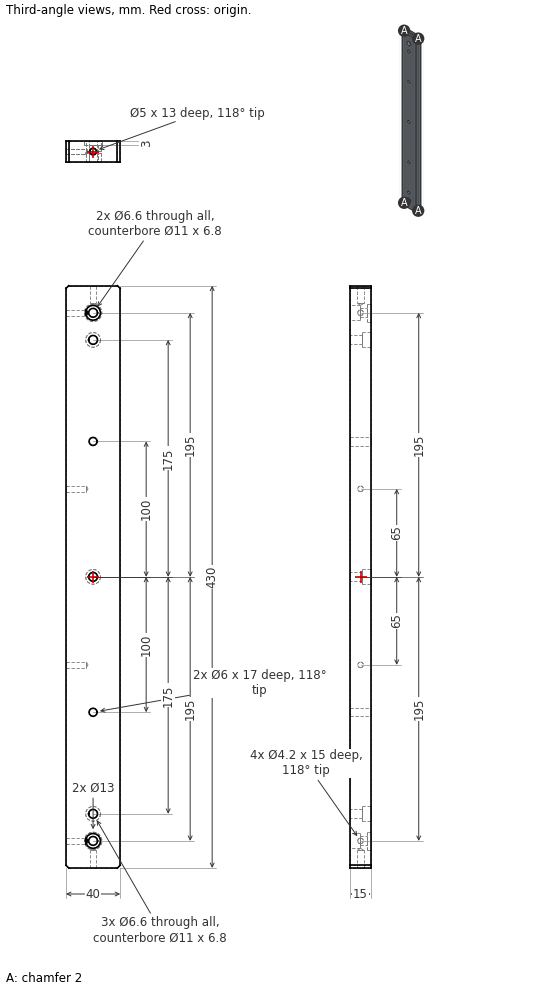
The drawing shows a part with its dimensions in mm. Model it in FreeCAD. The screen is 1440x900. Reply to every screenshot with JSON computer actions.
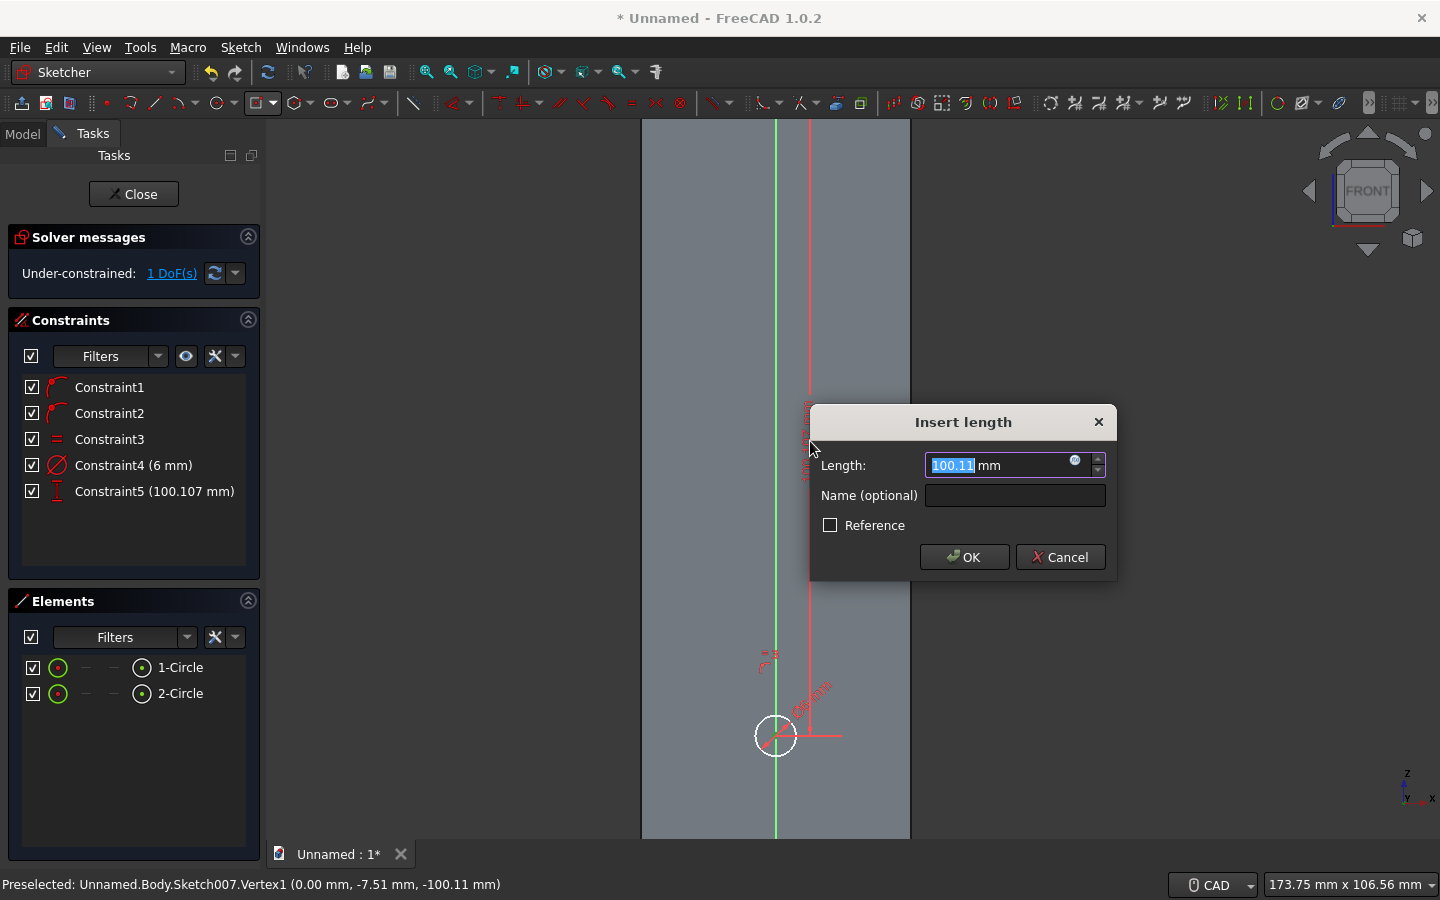
{"action": "type", "text": "100"}
{"action": "key", "text": "Return"}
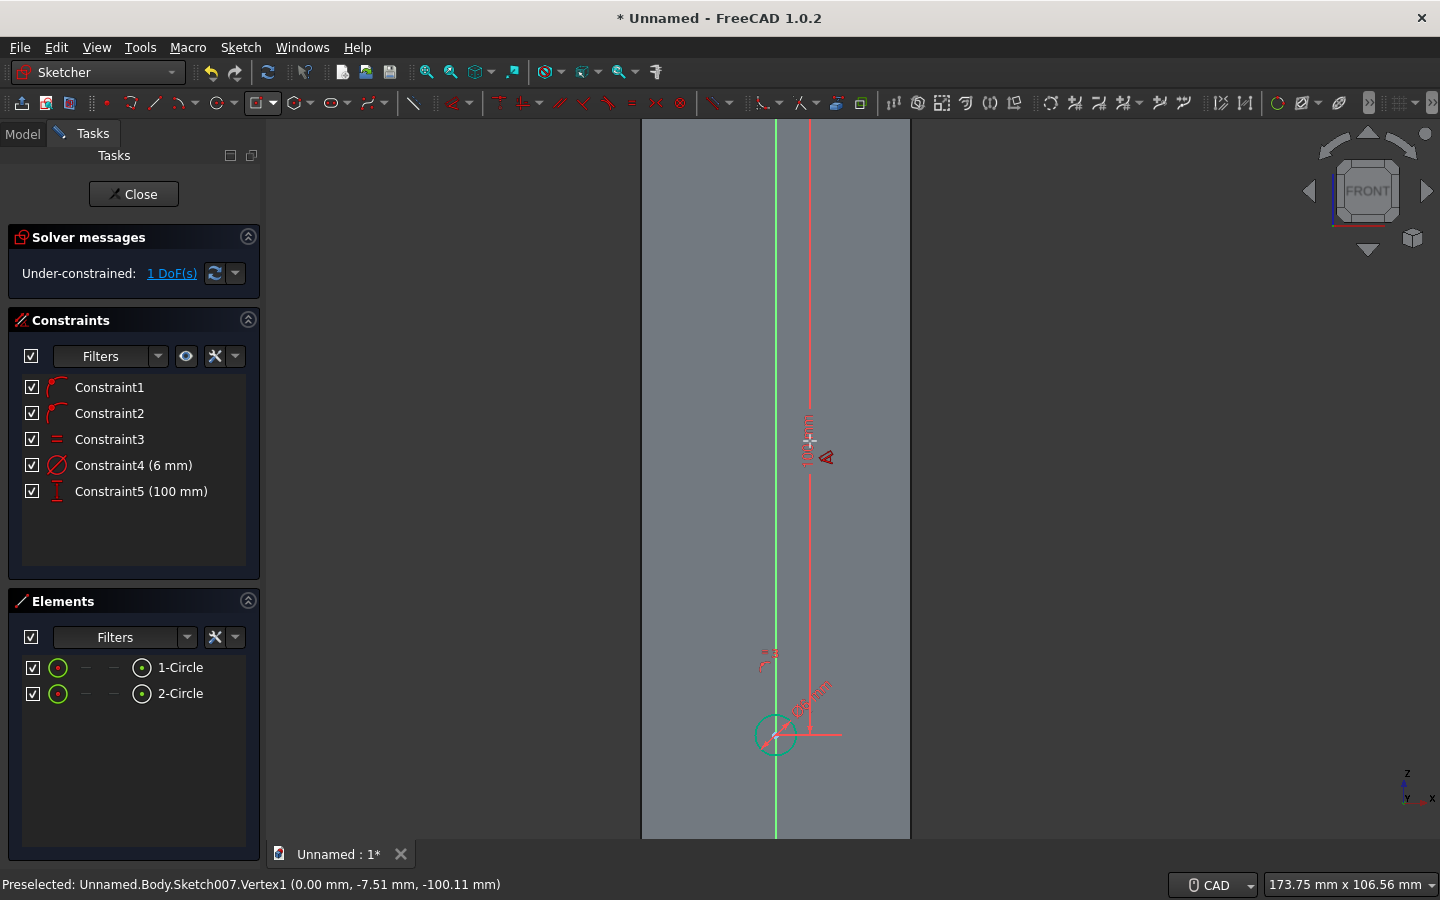
{"action": "scroll", "coordinate": [790, 723], "scroll_direction": "down", "scroll_amount": 5}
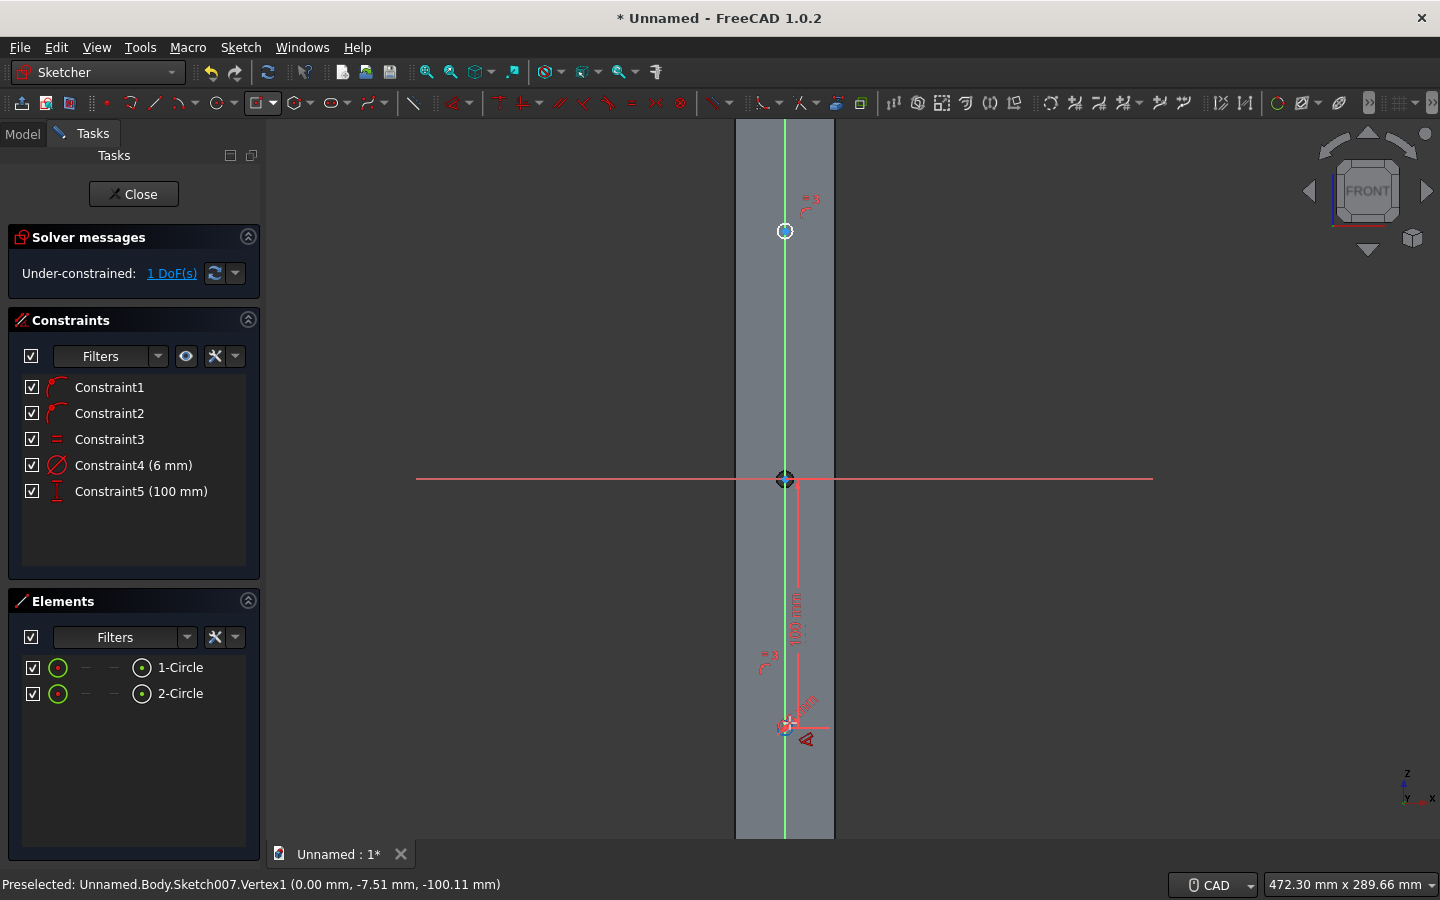
{"action": "left_click", "coordinate": [785, 231]}
{"action": "left_click", "coordinate": [819, 355]}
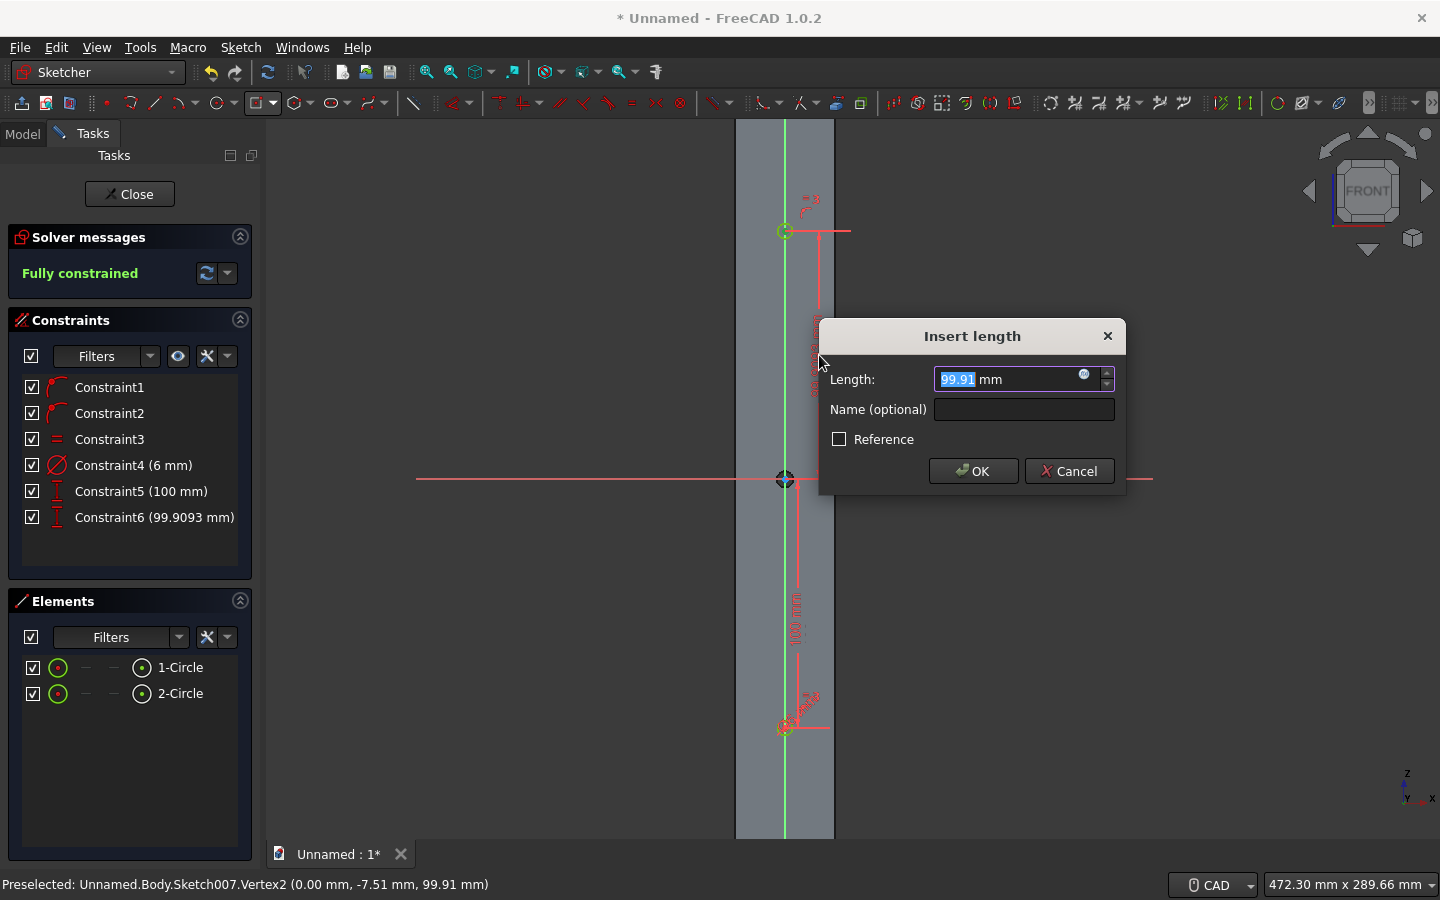
{"action": "type", "text": "100"}
{"action": "key", "text": "Return"}
{"action": "key", "text": "Escape"}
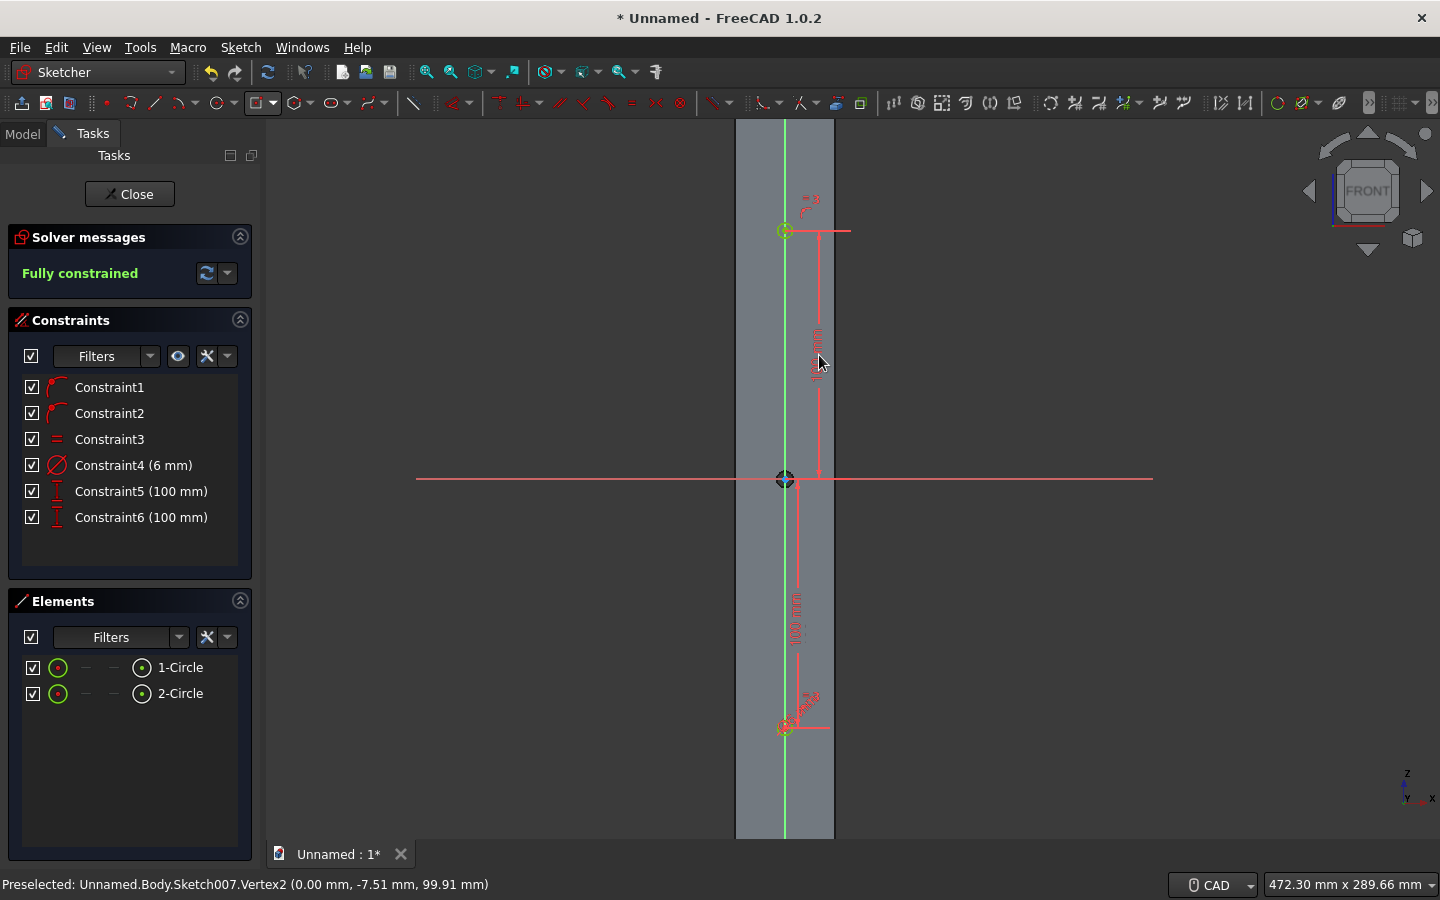
{"action": "left_click", "coordinate": [130, 194]}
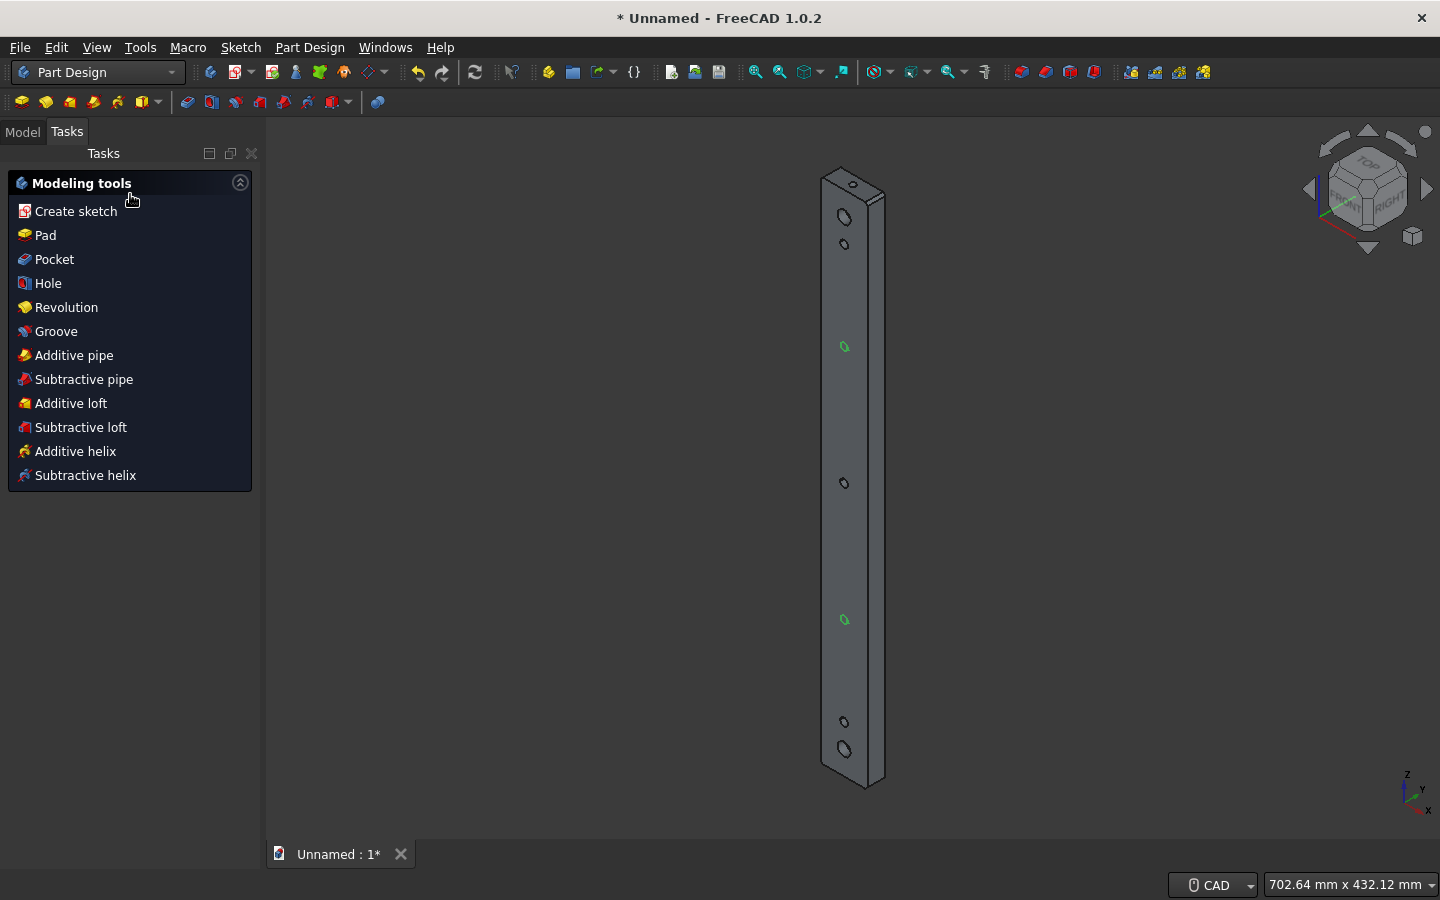
{"action": "left_click", "coordinate": [212, 102]}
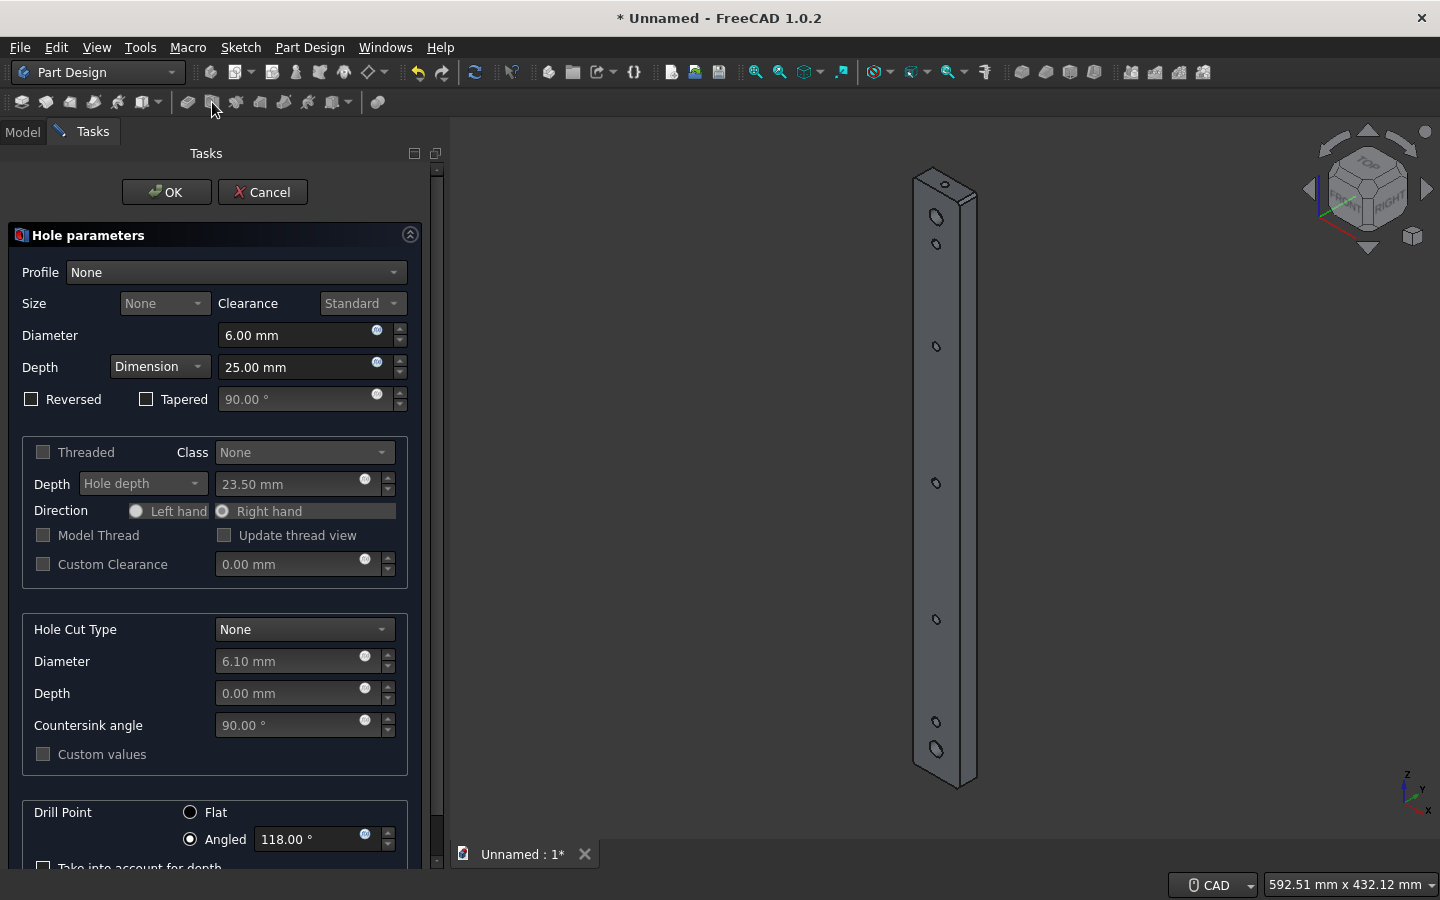
{"action": "triple_click", "coordinate": [305, 335]}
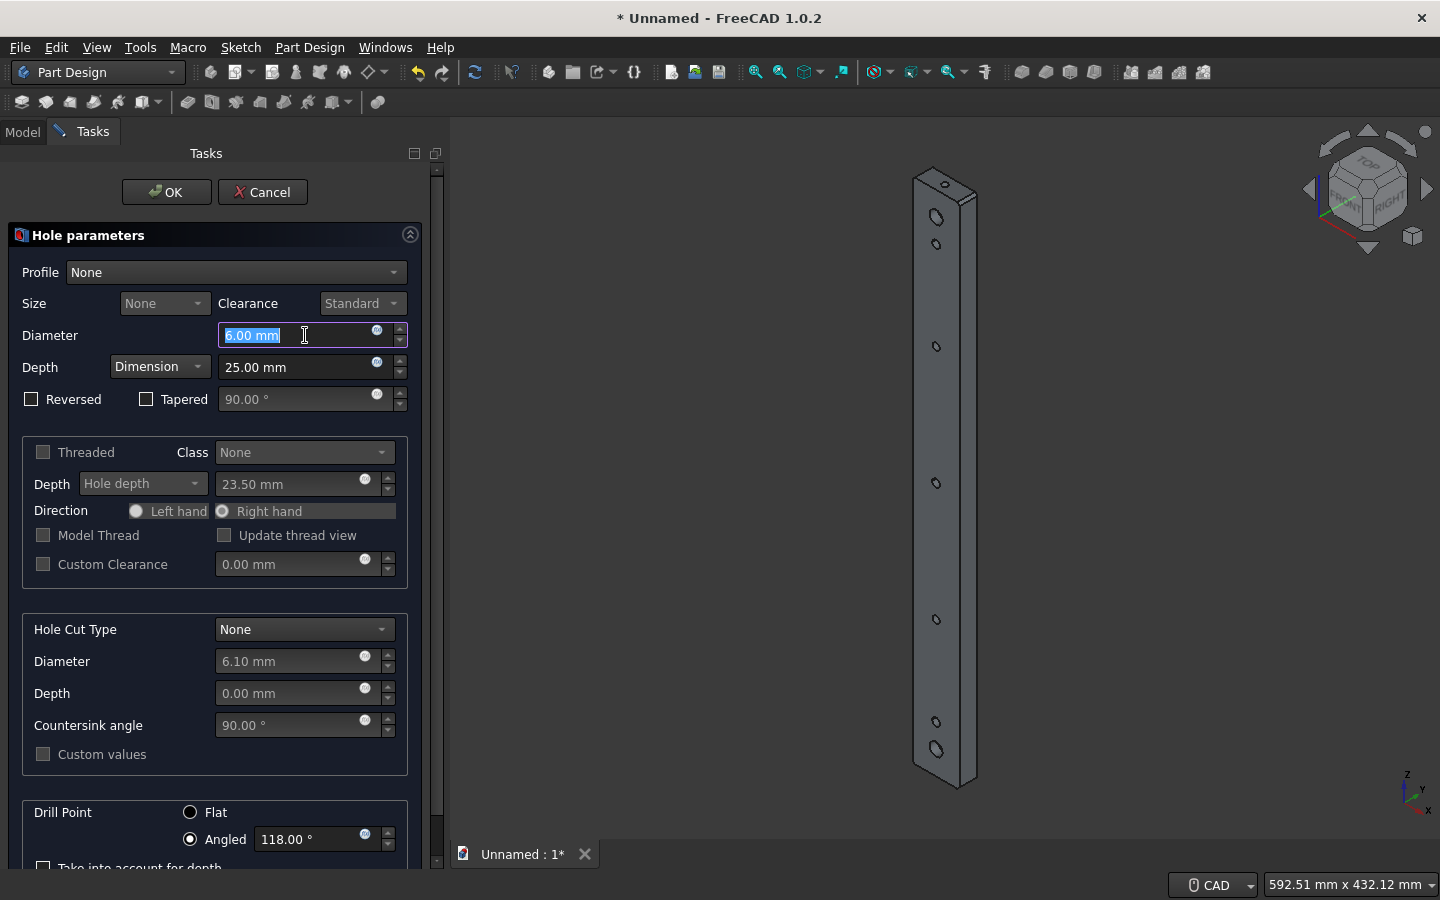
{"action": "type", "text": "6"}
{"action": "key", "text": "Tab"}